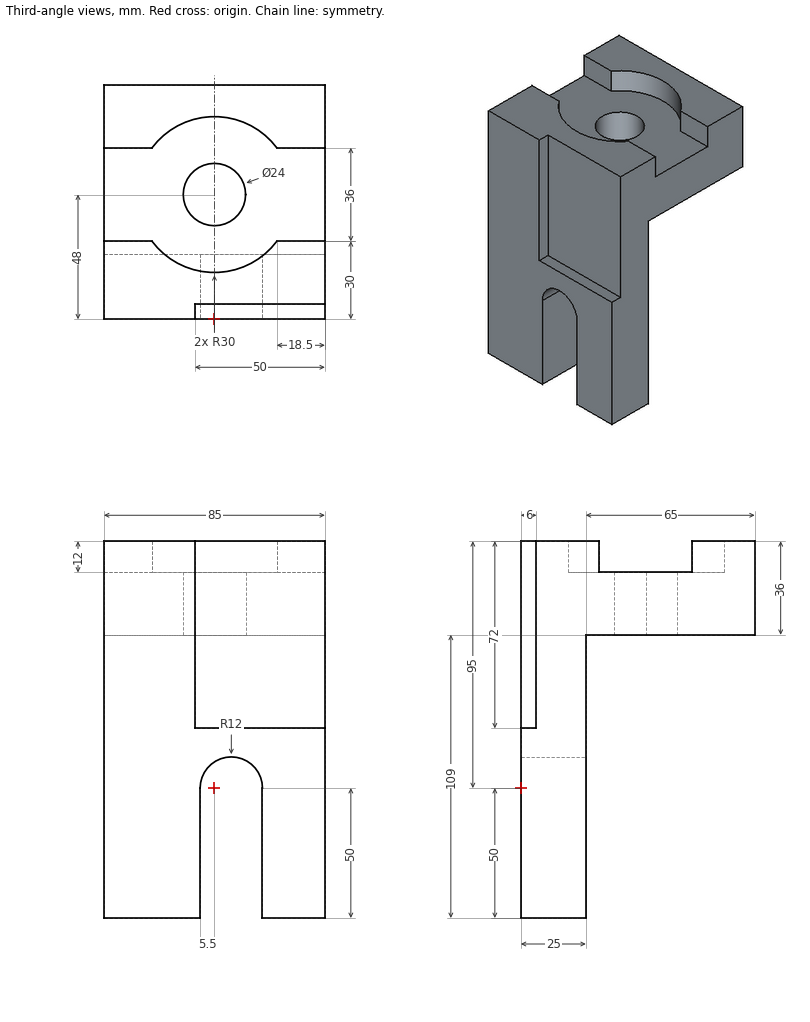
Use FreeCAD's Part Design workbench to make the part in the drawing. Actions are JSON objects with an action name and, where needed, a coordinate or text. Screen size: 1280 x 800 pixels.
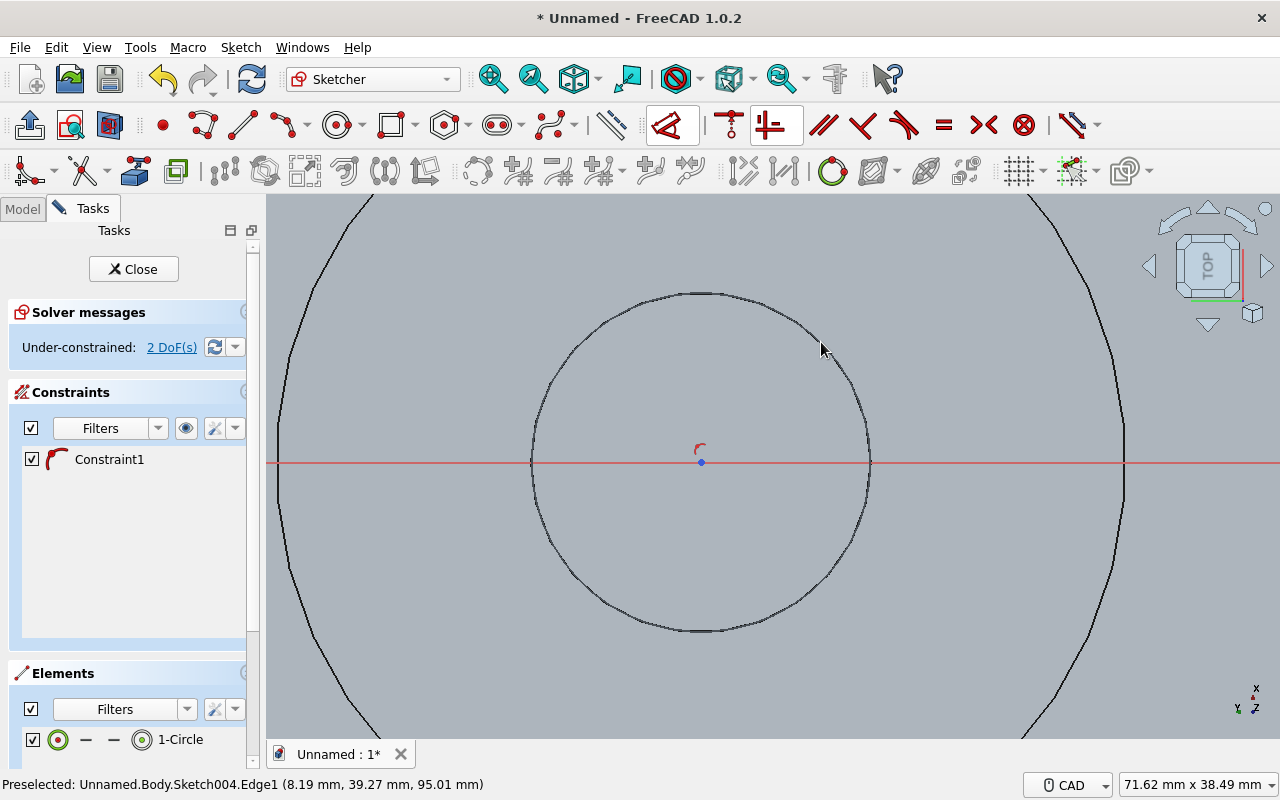
{"action": "left_click", "coordinate": [820, 342]}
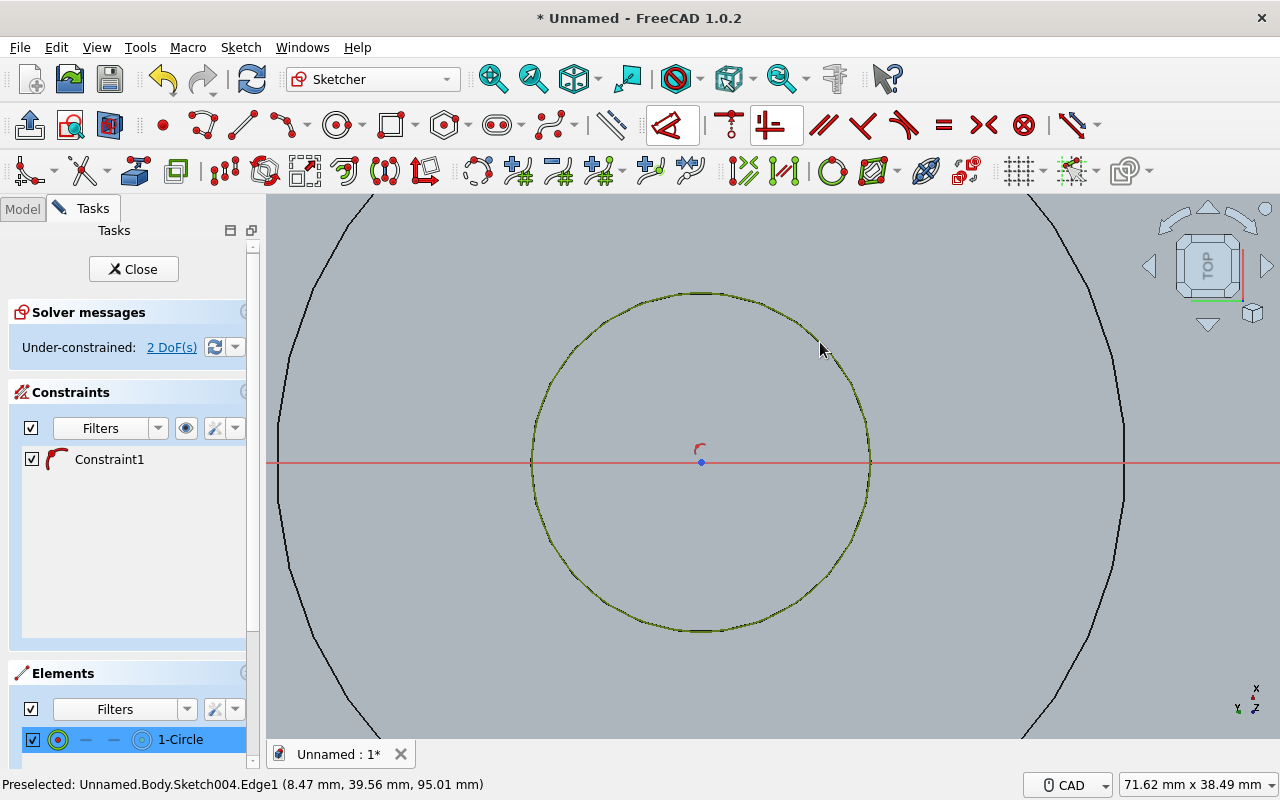
{"action": "key", "text": "k o"}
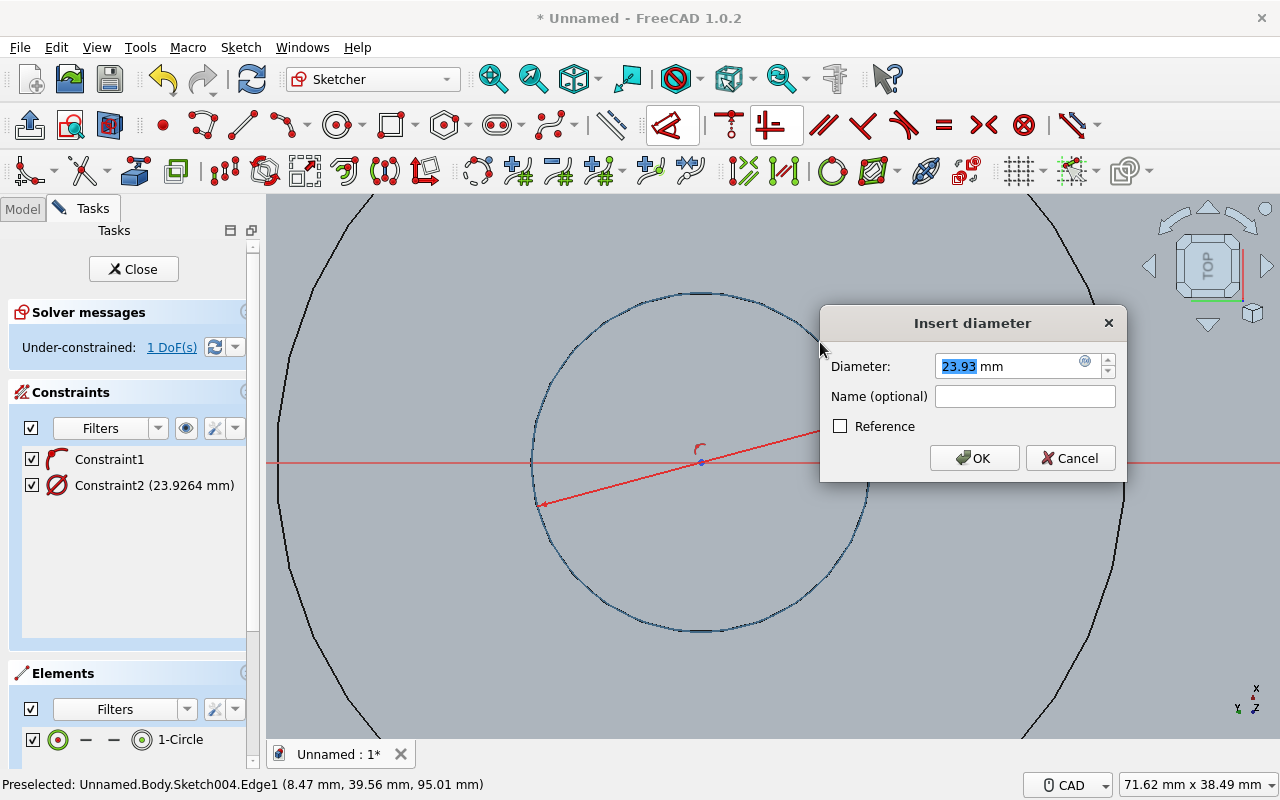
{"action": "type", "text": "24"}
{"action": "key", "text": "Return"}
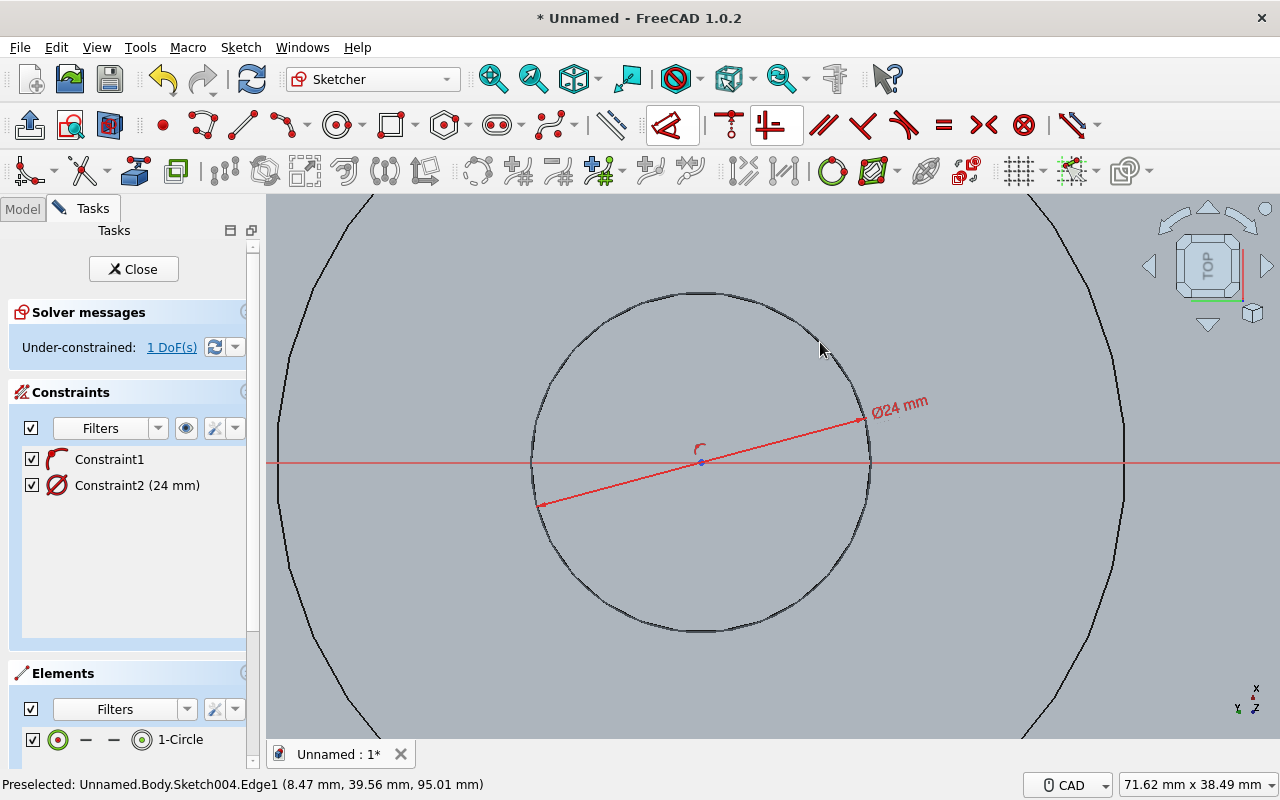
{"action": "left_click", "coordinate": [701, 463]}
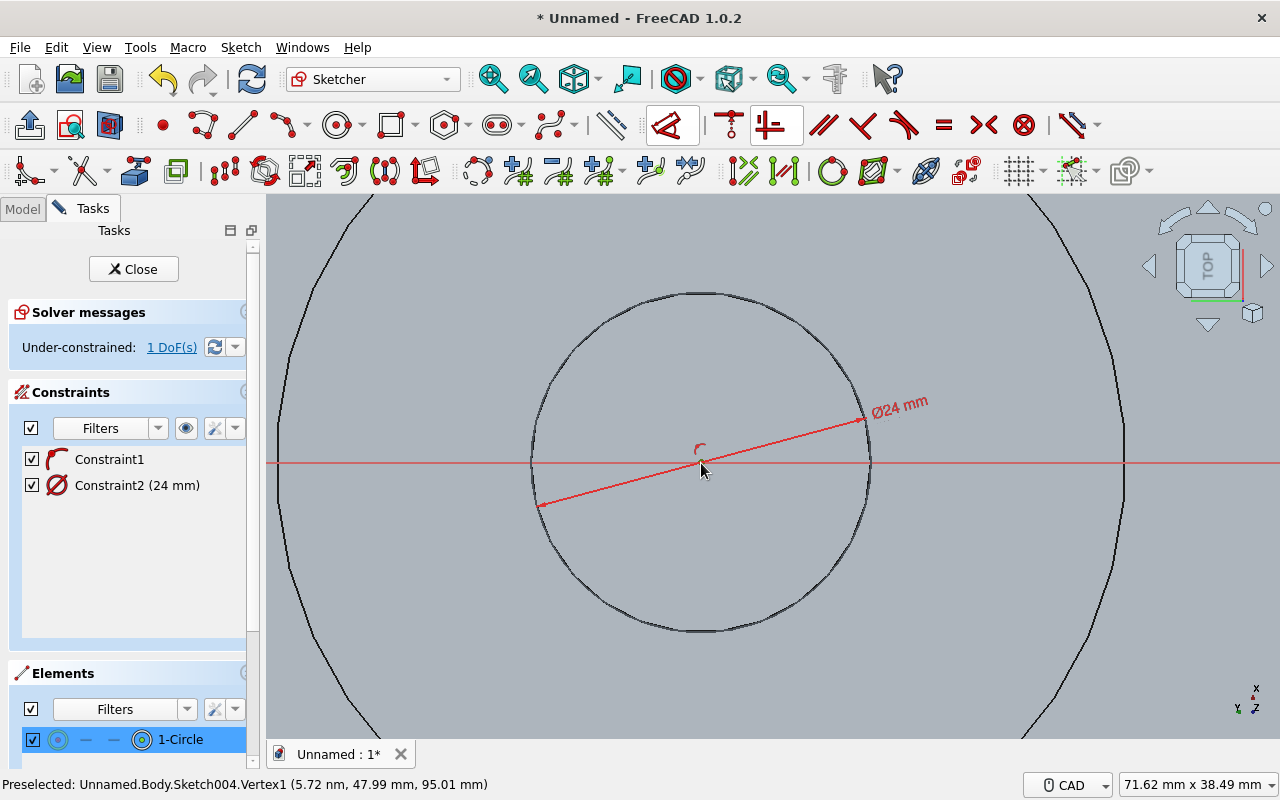
{"action": "key", "text": "l"}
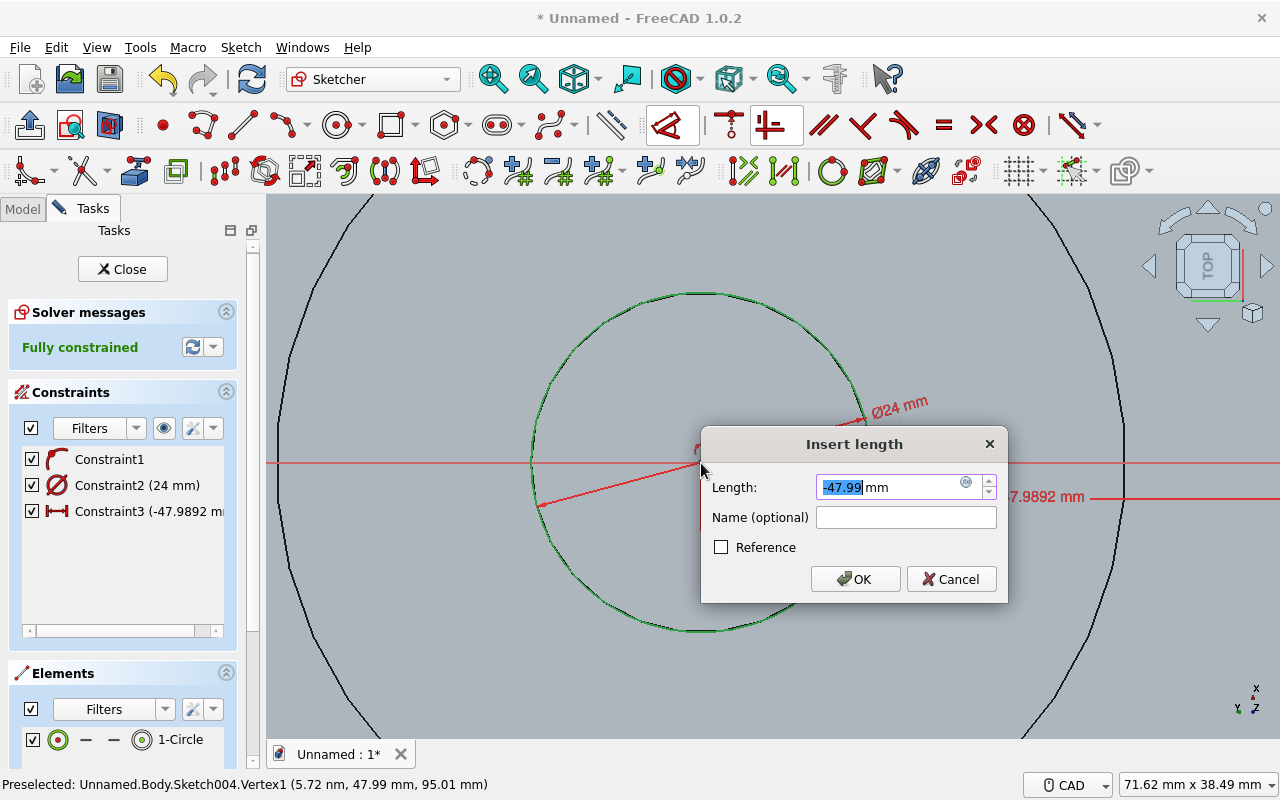
{"action": "type", "text": "-48"}
{"action": "key", "text": "Return"}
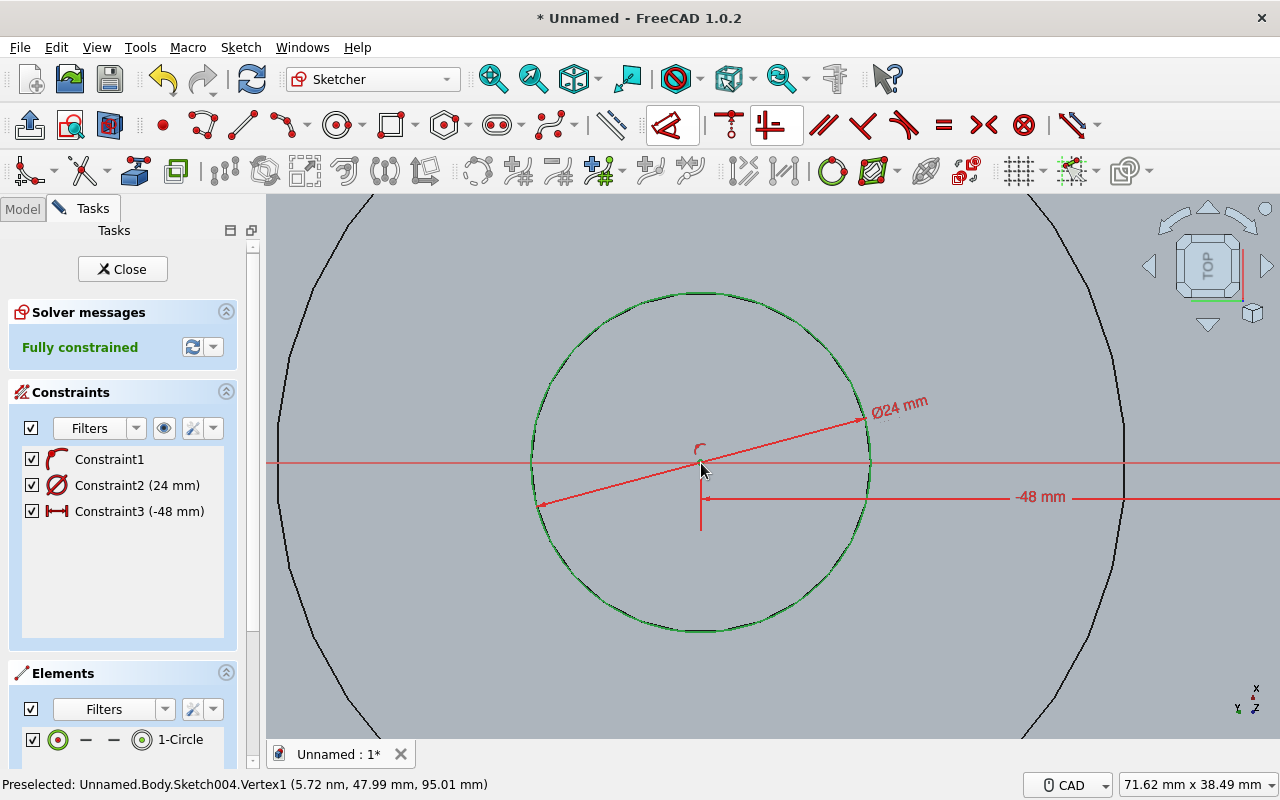
{"action": "left_click", "coordinate": [123, 269]}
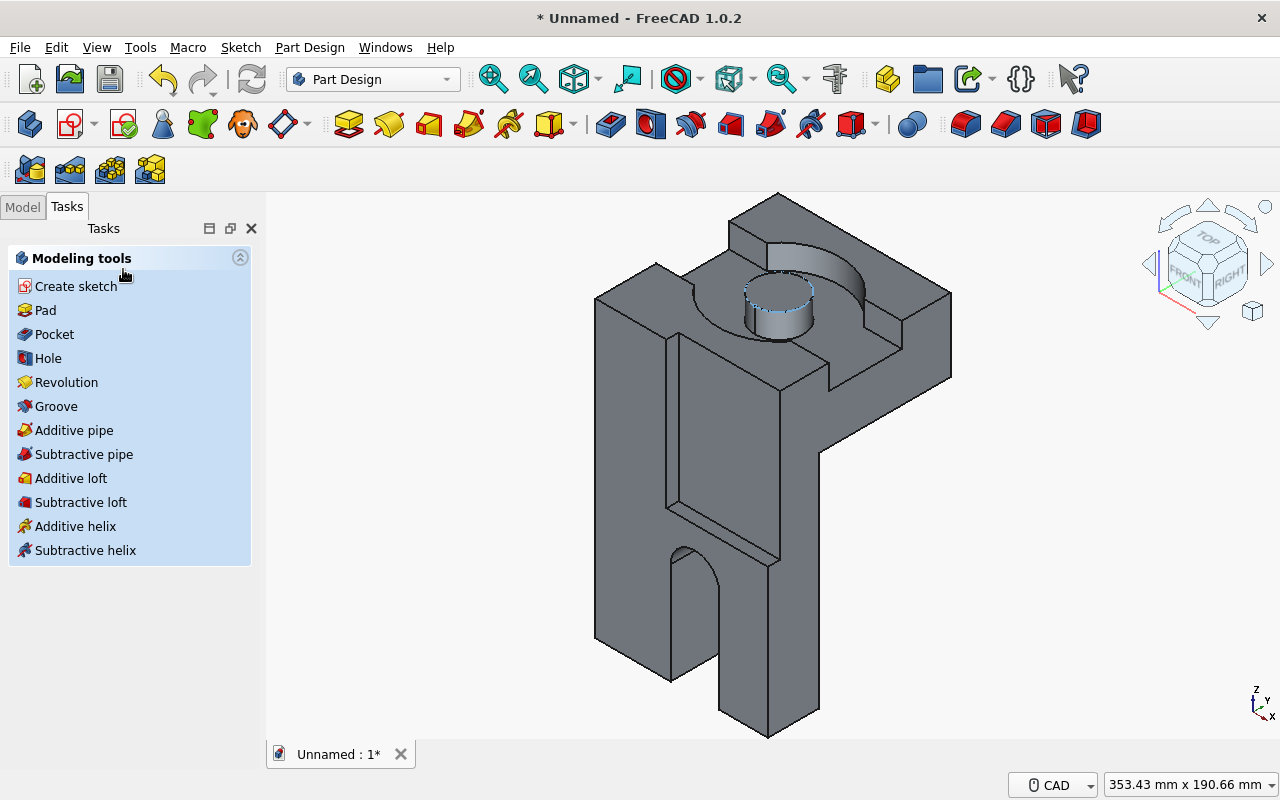
{"action": "left_click", "coordinate": [612, 124]}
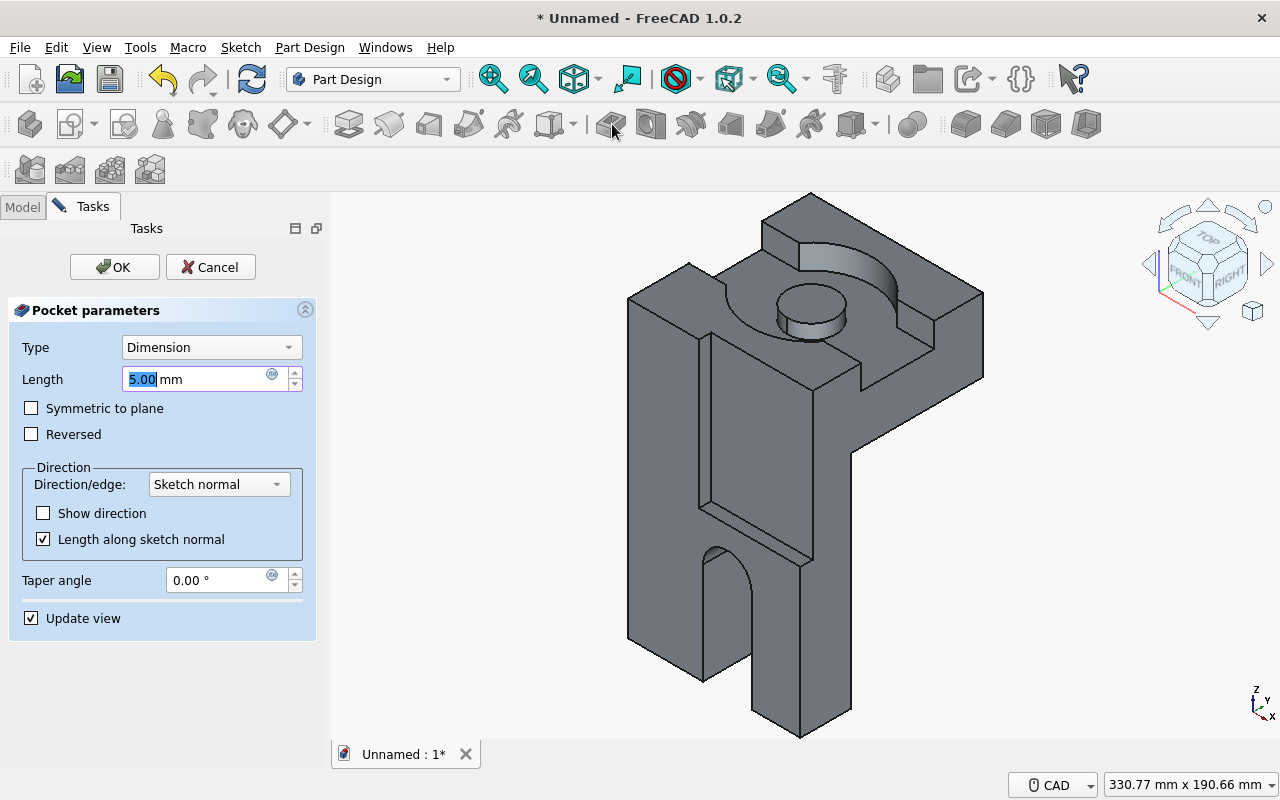
{"action": "left_click", "coordinate": [212, 348]}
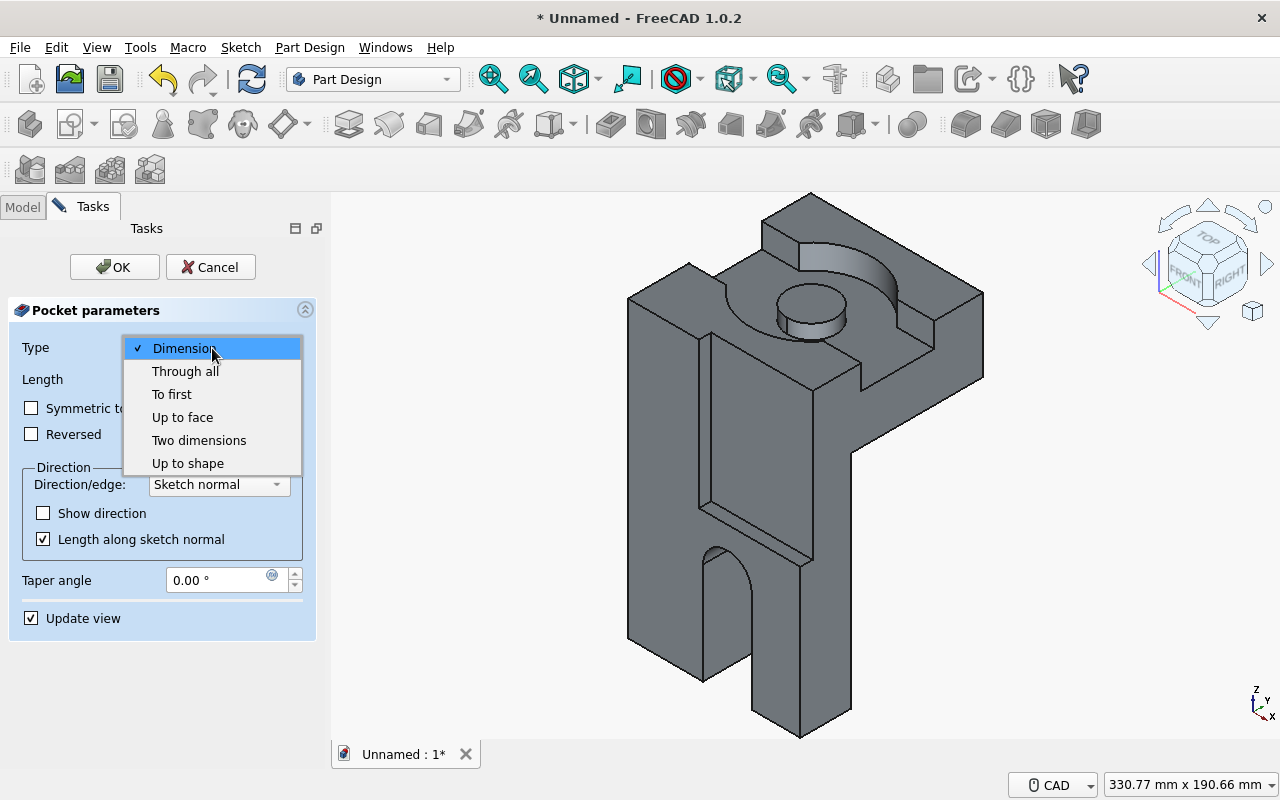
{"action": "left_click", "coordinate": [212, 394]}